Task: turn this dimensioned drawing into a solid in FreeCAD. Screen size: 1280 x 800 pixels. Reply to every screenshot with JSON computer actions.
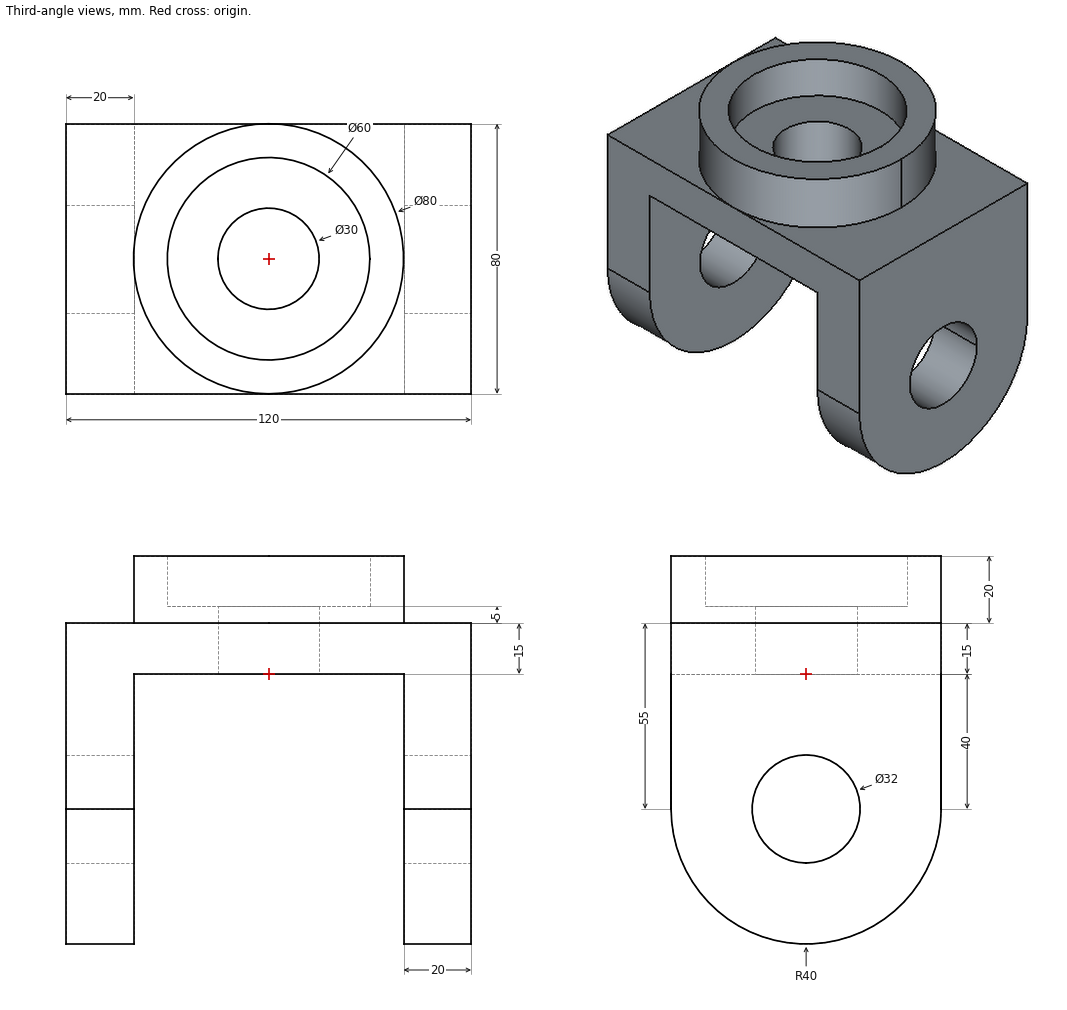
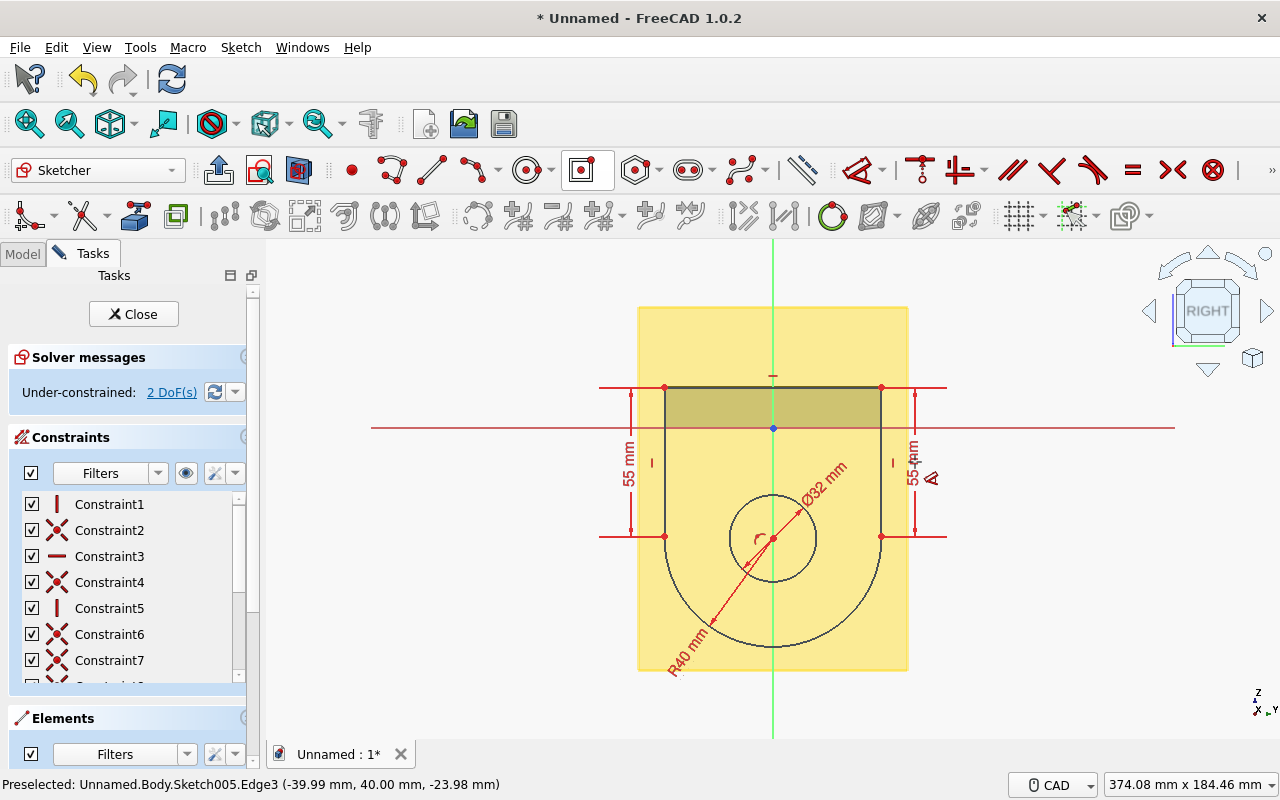
{"action": "left_click", "coordinate": [773, 538]}
{"action": "left_click", "coordinate": [807, 458]}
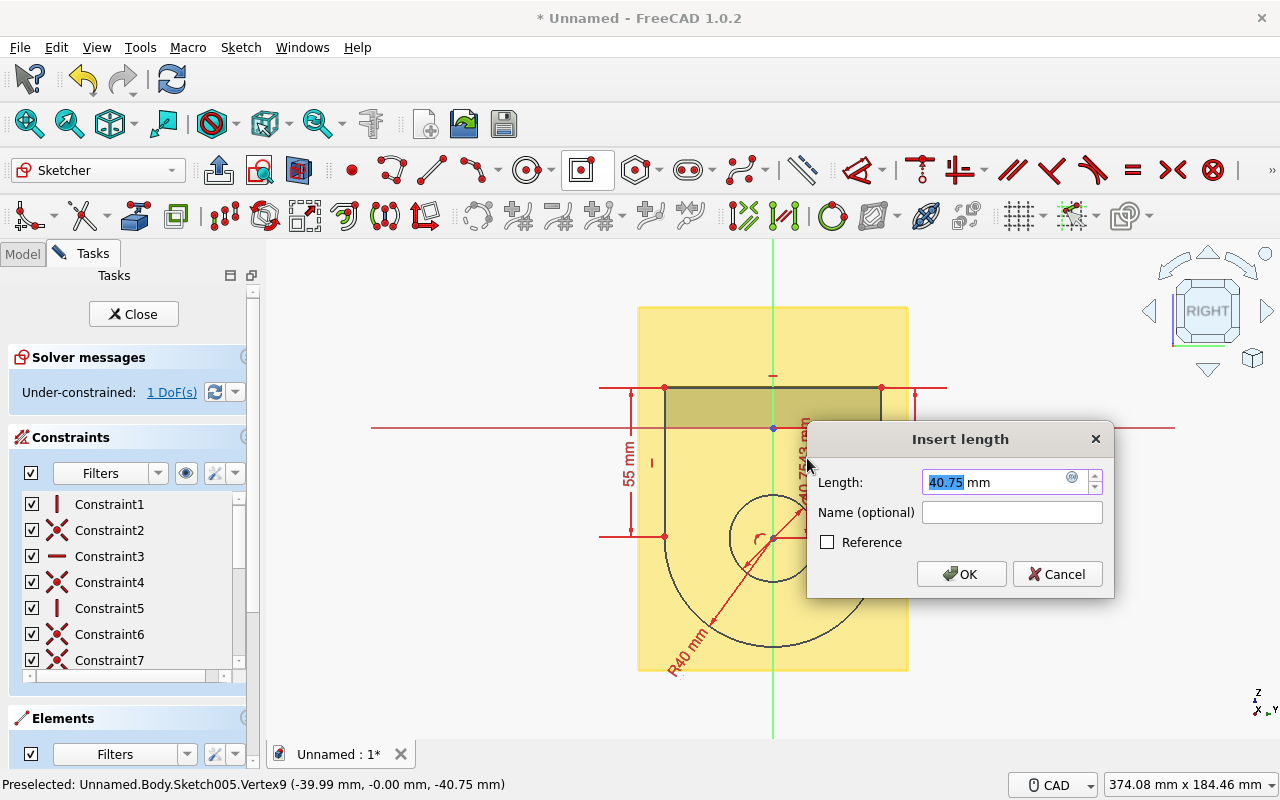
{"action": "type", "text": "40"}
{"action": "key", "text": "Return"}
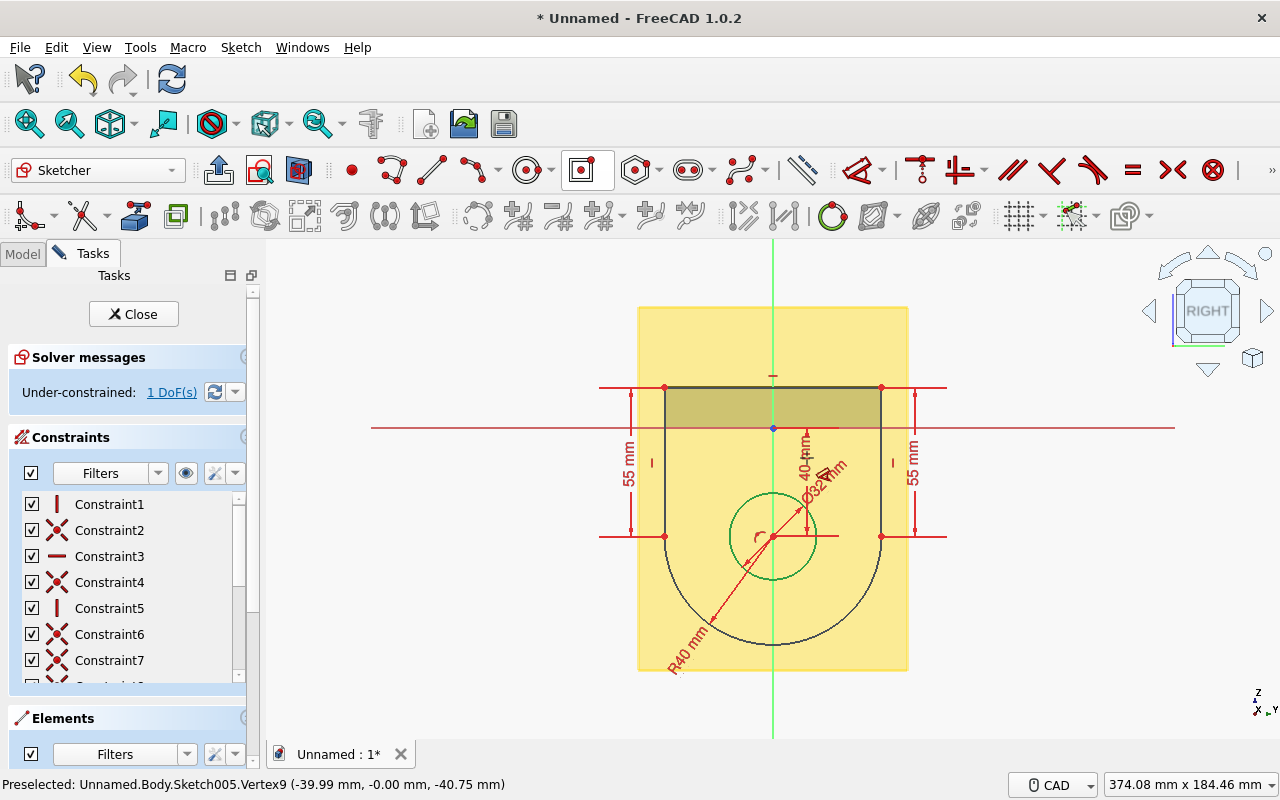
{"action": "left_click", "coordinate": [665, 537]}
{"action": "left_click", "coordinate": [631, 483]}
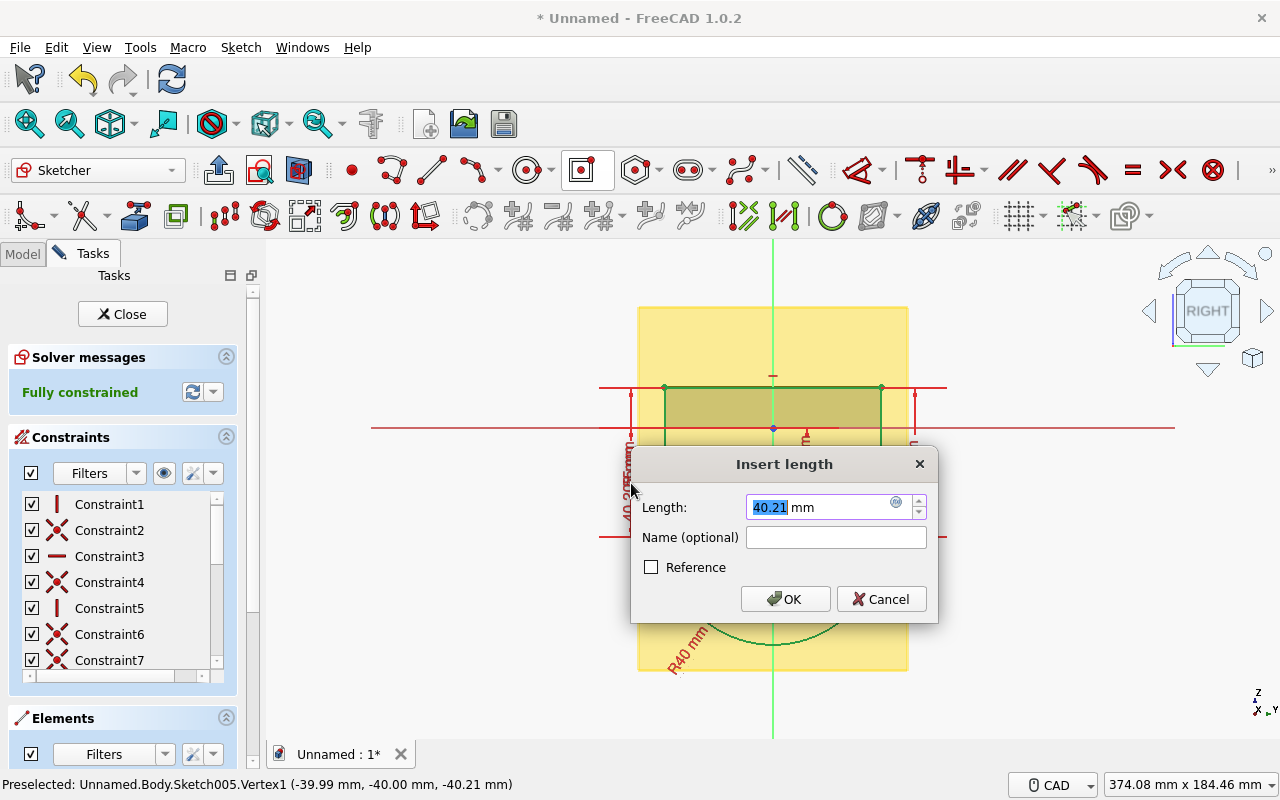
{"action": "type", "text": "40"}
{"action": "key", "text": "Return"}
{"action": "key", "text": "Escape"}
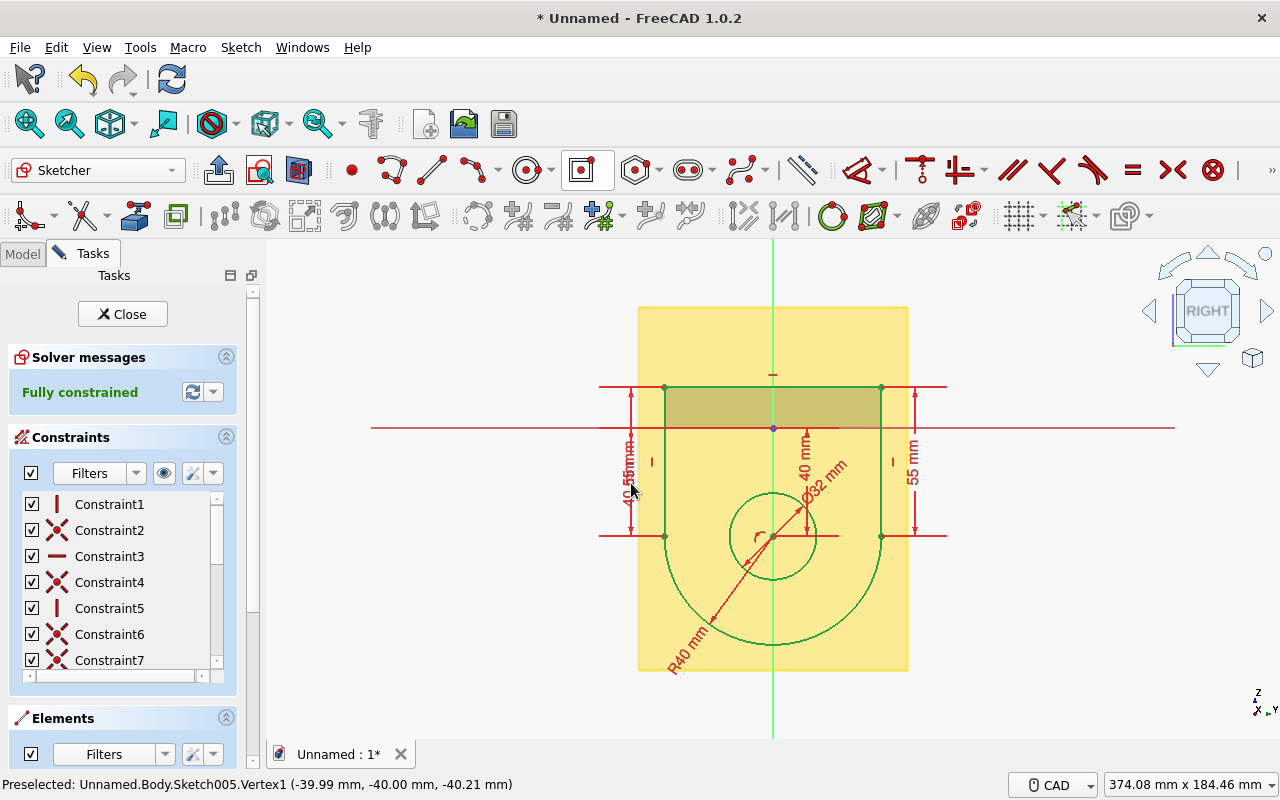
{"action": "left_click", "coordinate": [123, 314]}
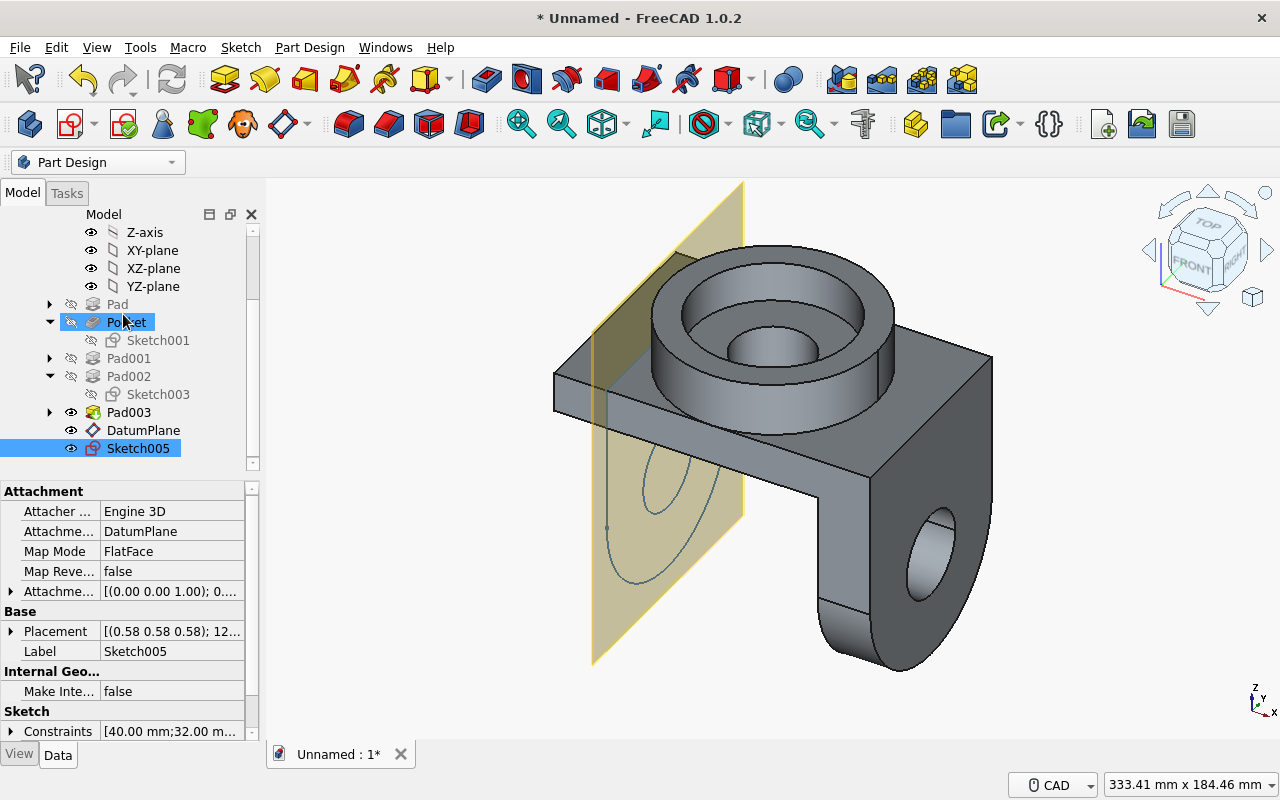
{"action": "left_click", "coordinate": [226, 80]}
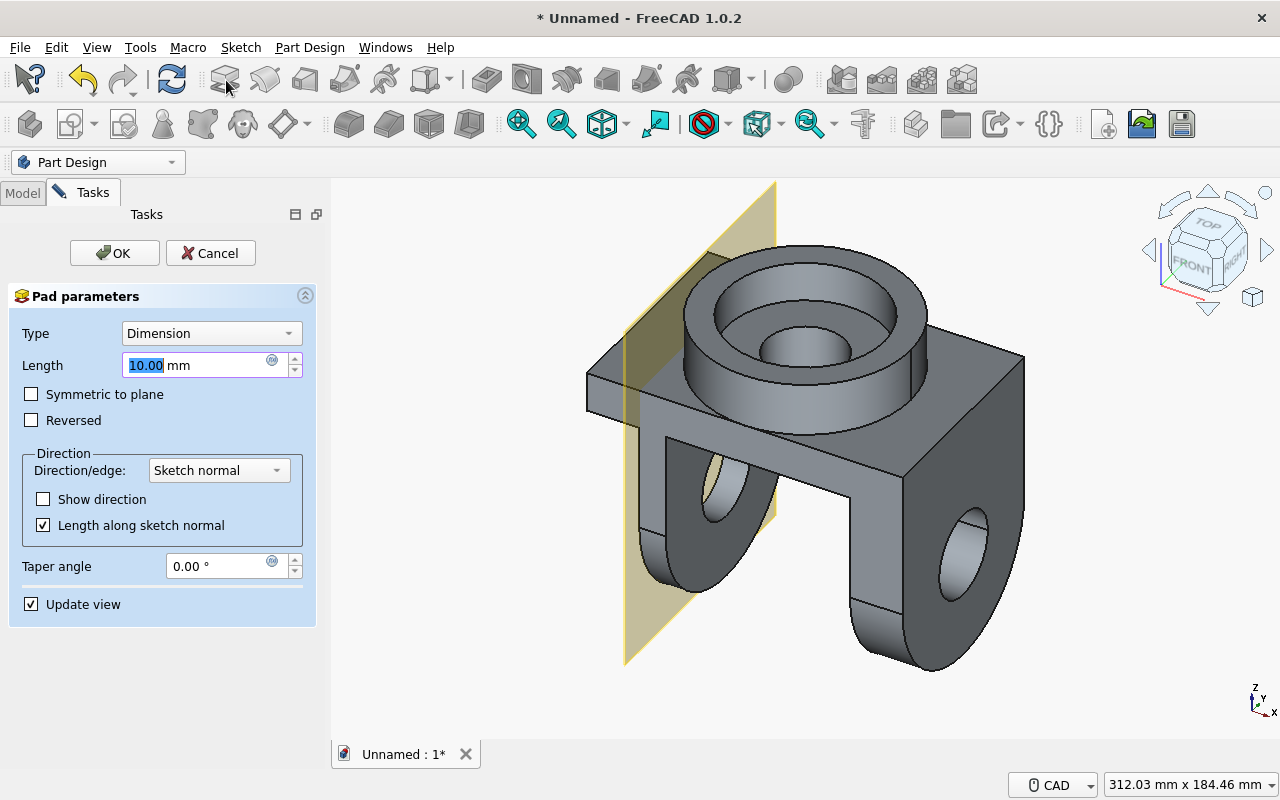
{"action": "type", "text": "20"}
{"action": "key", "text": "Tab"}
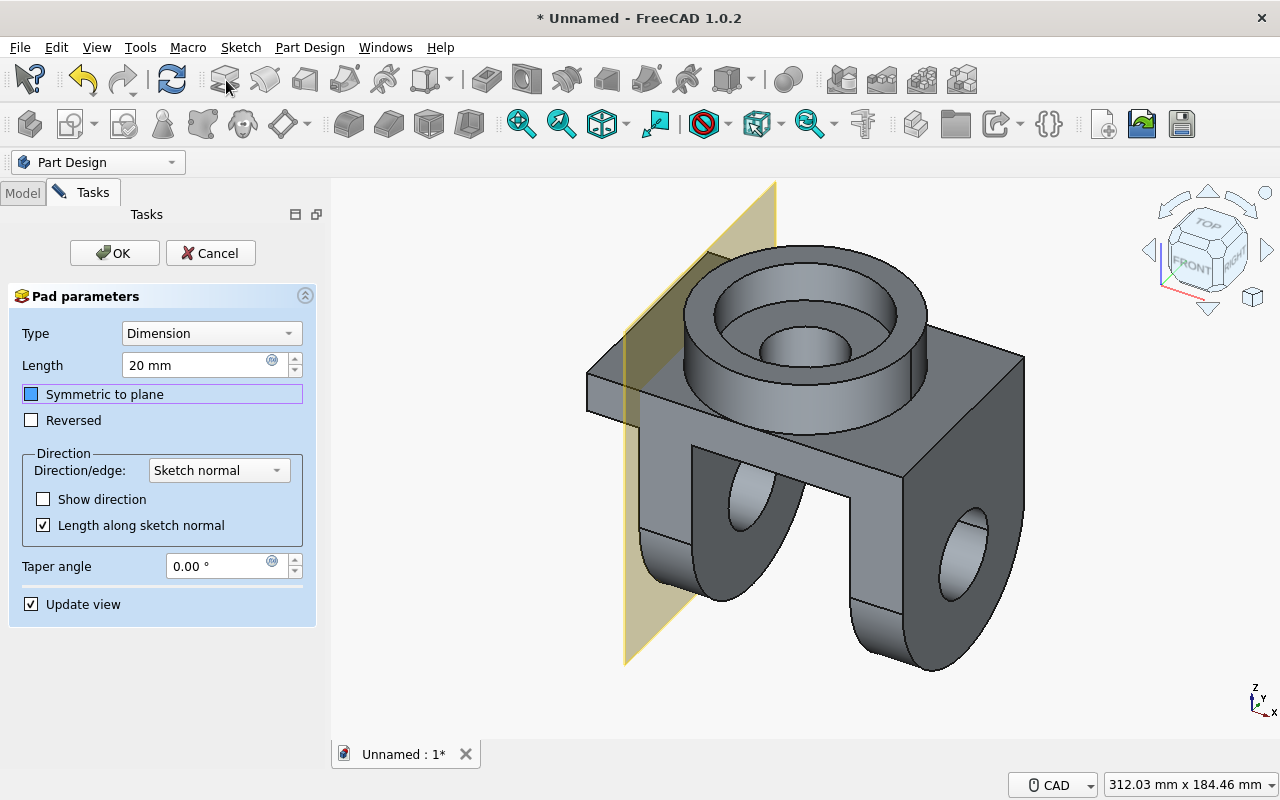
{"action": "left_click", "coordinate": [30, 420]}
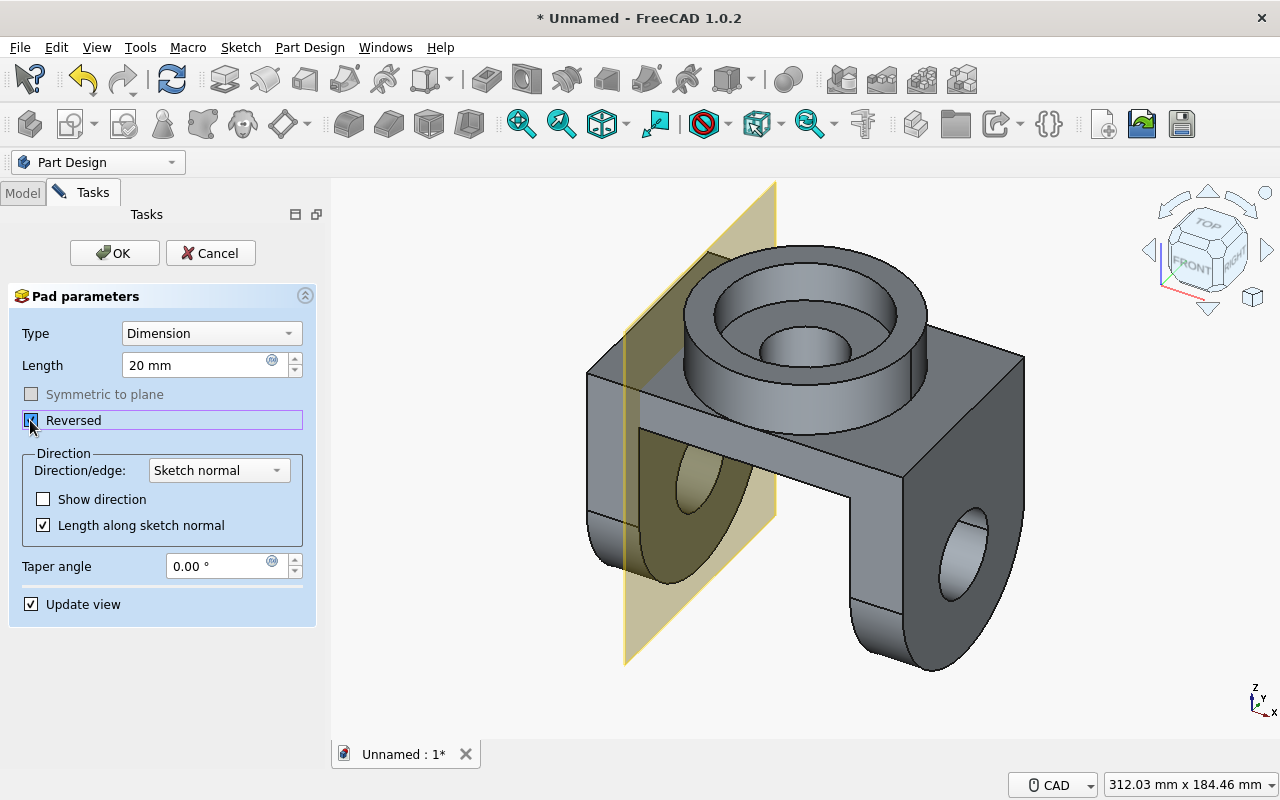
{"action": "left_click", "coordinate": [115, 253]}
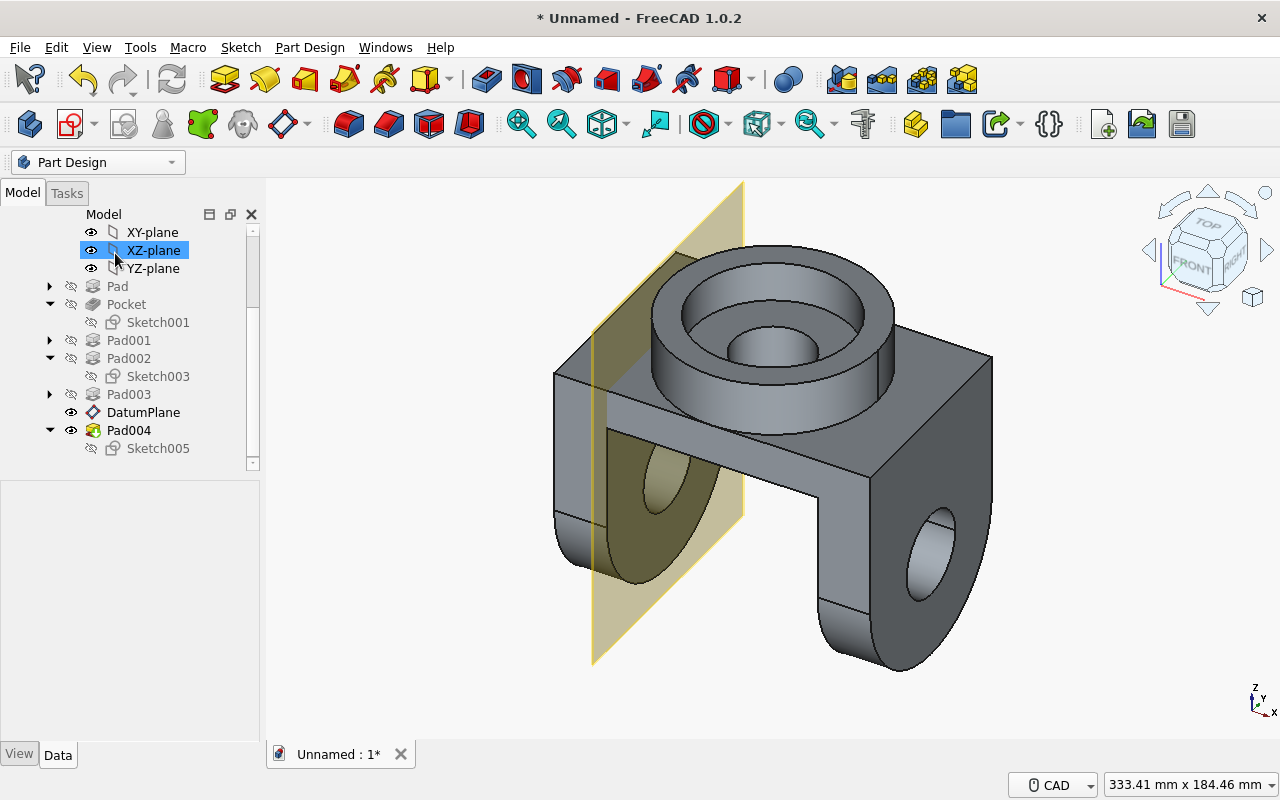
{"action": "left_click", "coordinate": [116, 412]}
{"action": "key", "text": "space"}